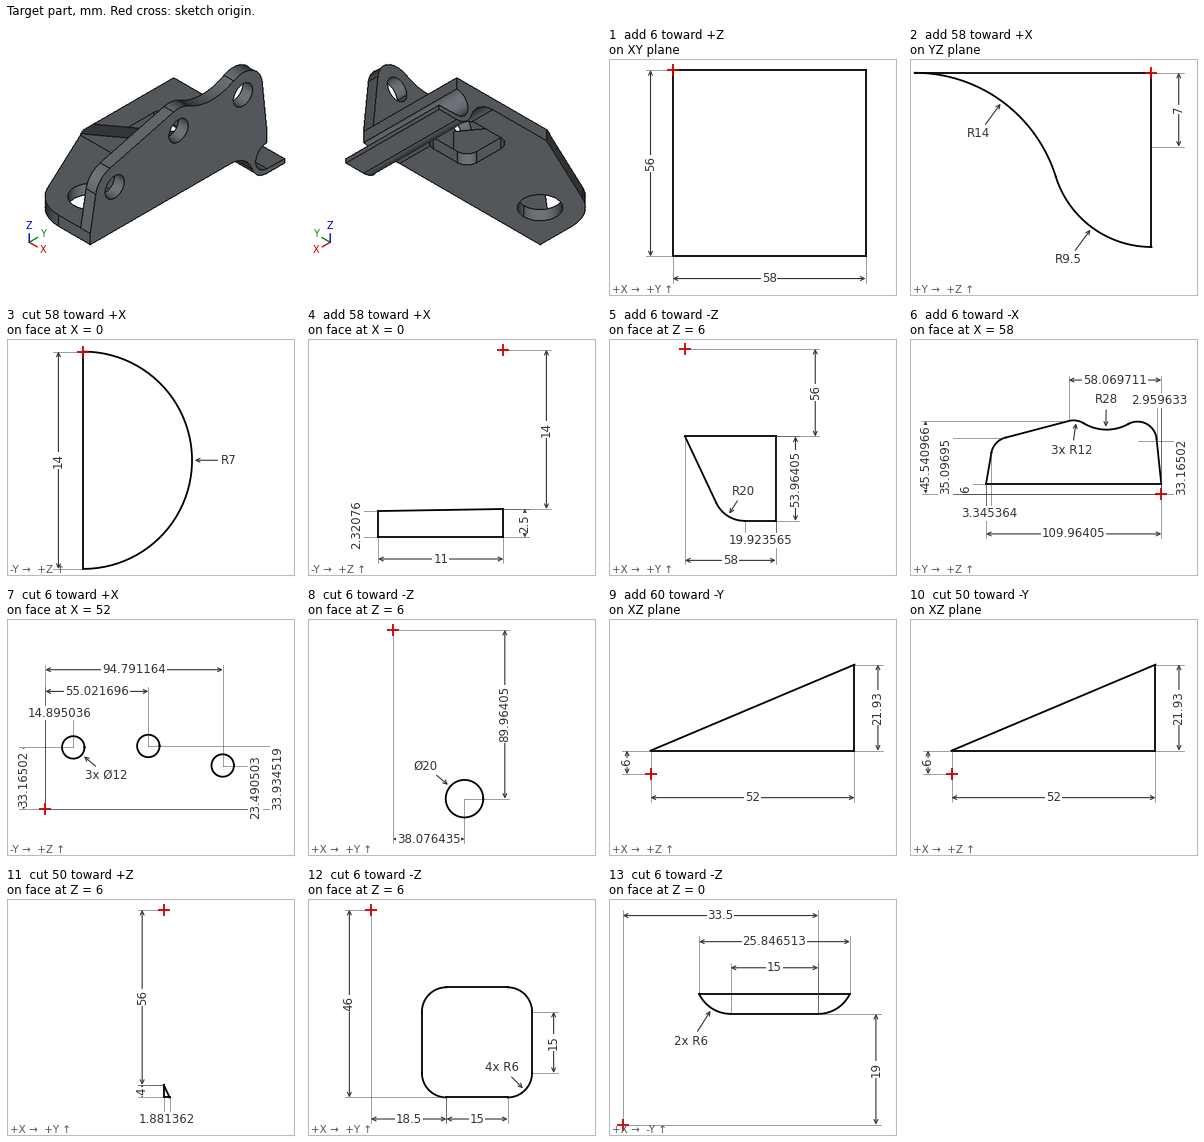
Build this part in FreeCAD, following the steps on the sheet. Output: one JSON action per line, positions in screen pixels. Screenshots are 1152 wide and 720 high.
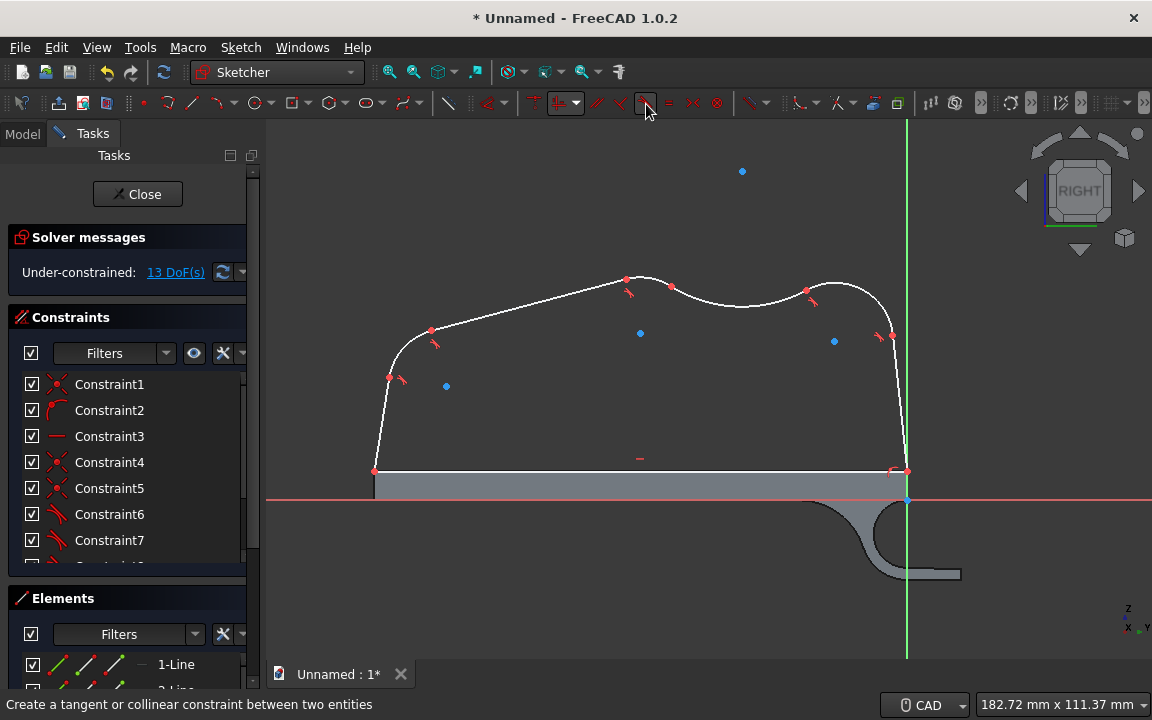
{"action": "left_click", "coordinate": [710, 303]}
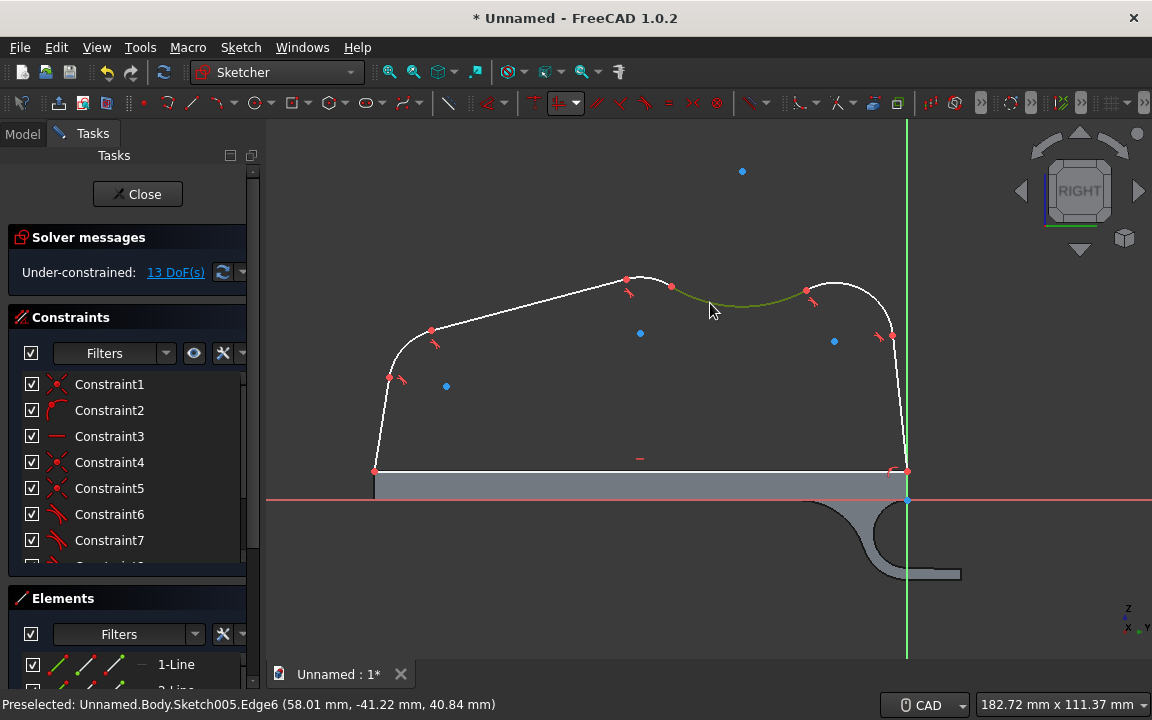
{"action": "left_click", "coordinate": [658, 280]}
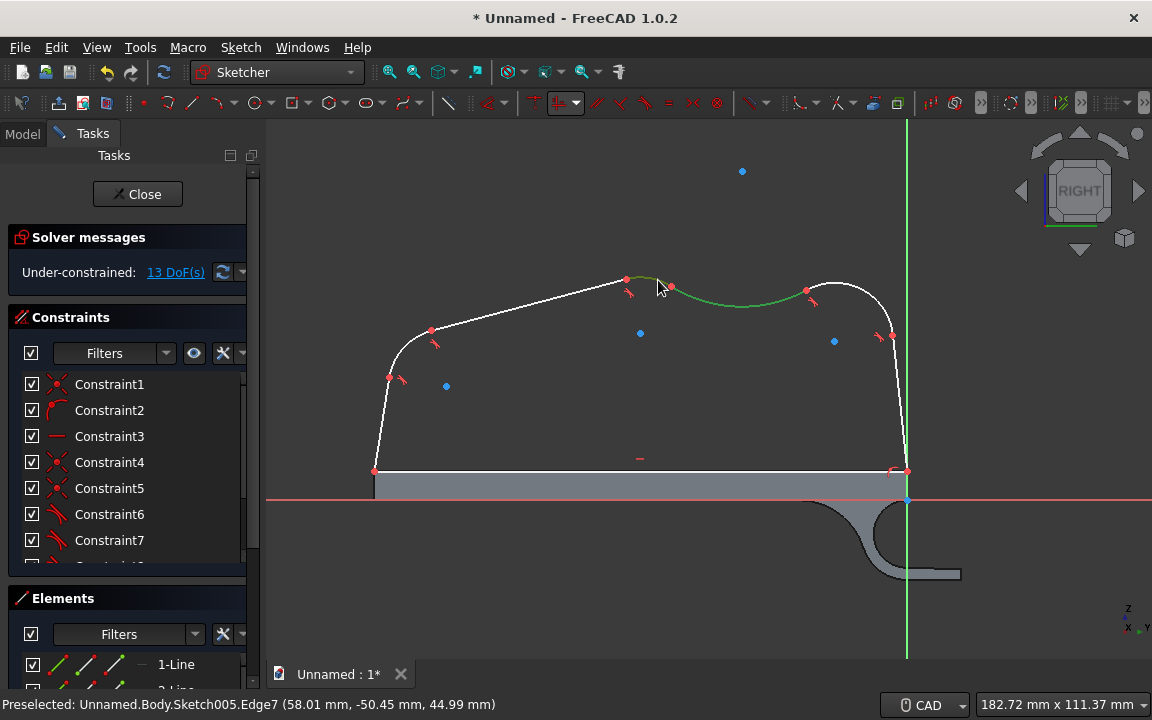
{"action": "key", "text": "t"}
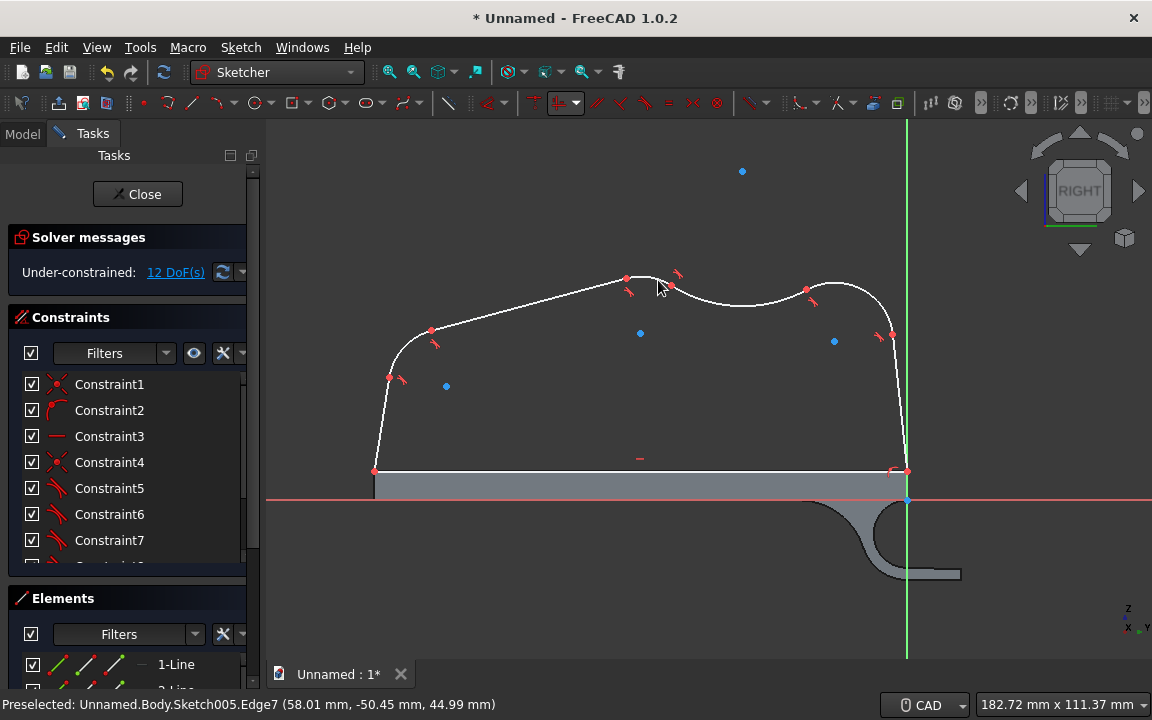
{"action": "left_click", "coordinate": [880, 304]}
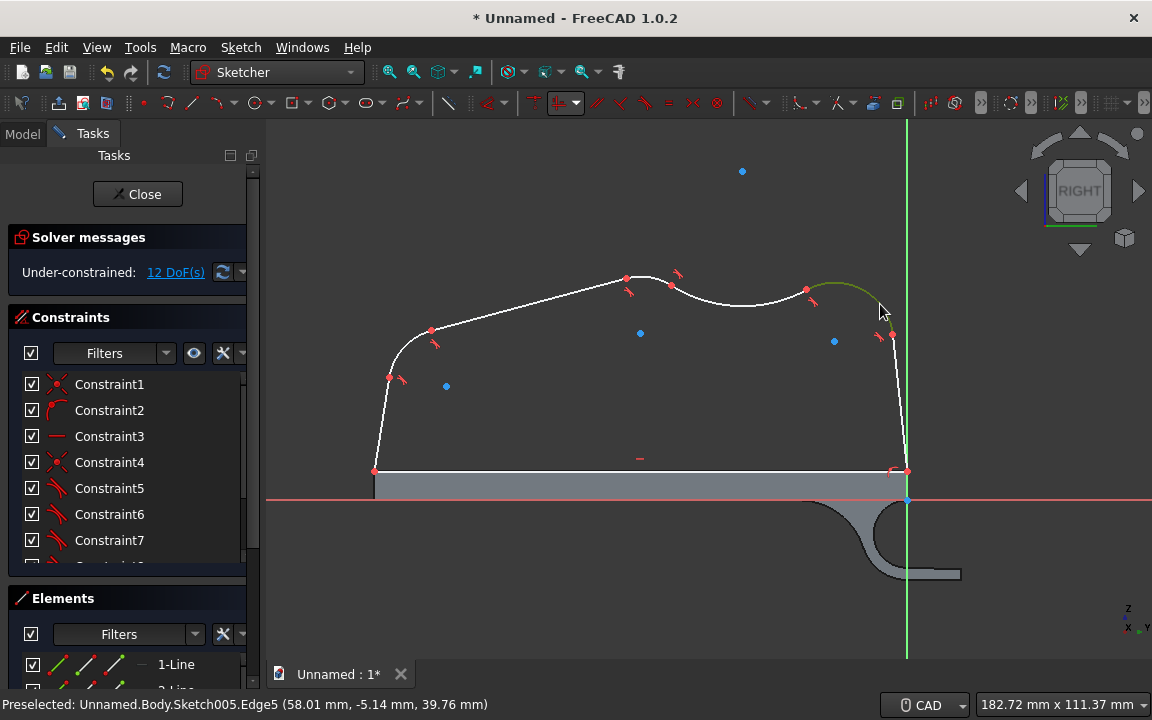
{"action": "left_click", "coordinate": [658, 279]}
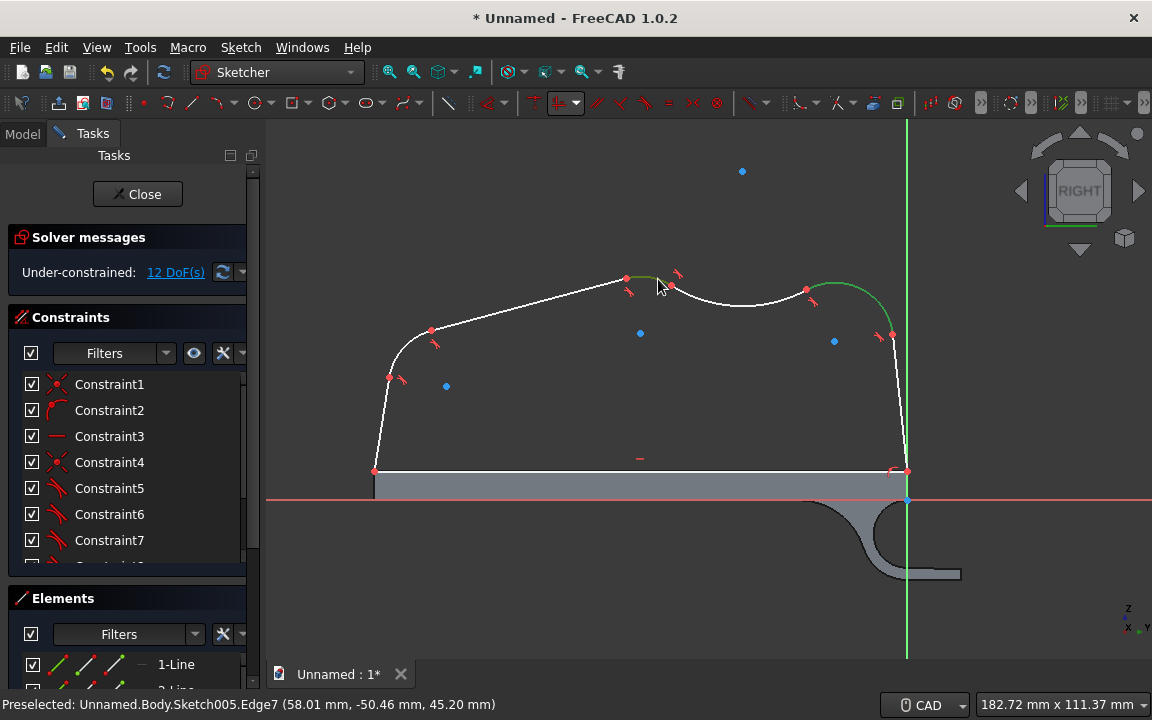
{"action": "left_click", "coordinate": [414, 339]}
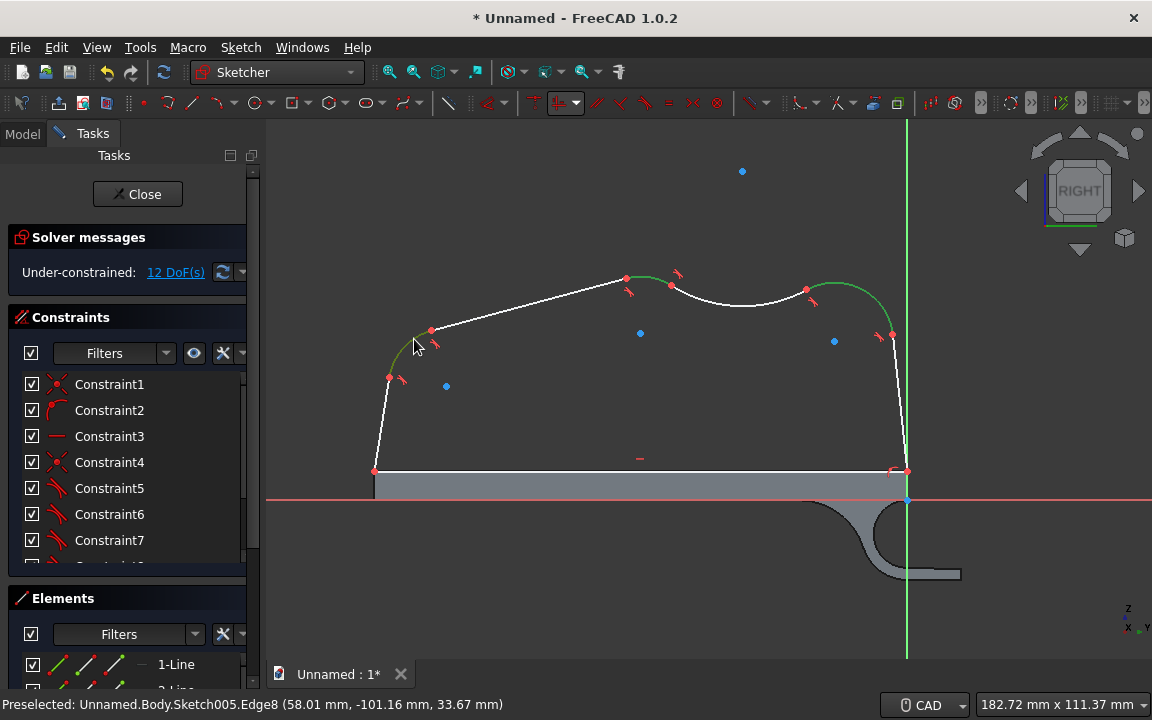
{"action": "left_click", "coordinate": [670, 104]}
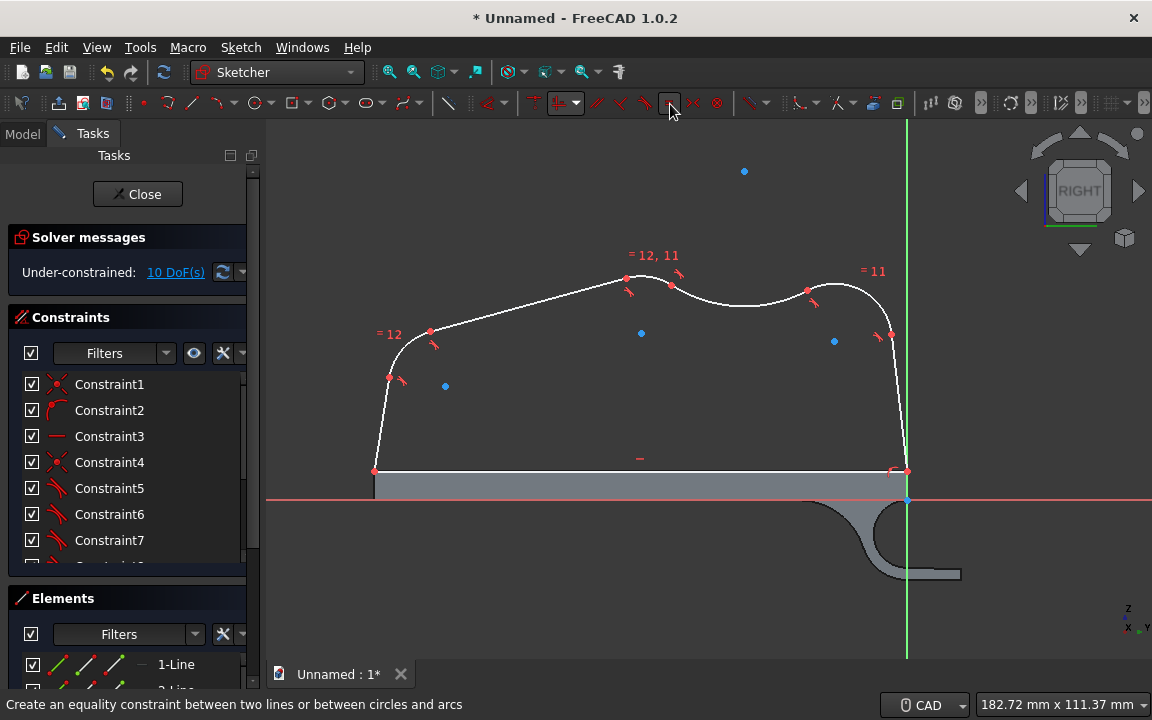
{"action": "left_click", "coordinate": [488, 104]}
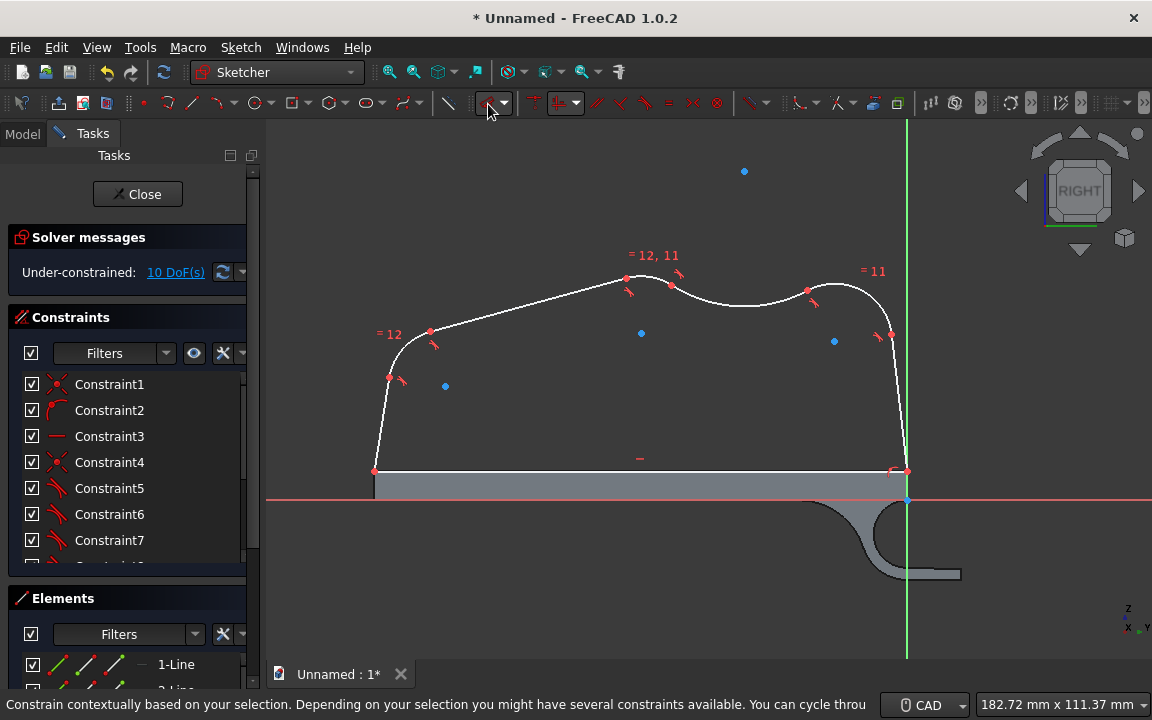
{"action": "left_click", "coordinate": [879, 304]}
{"action": "left_click", "coordinate": [923, 323]}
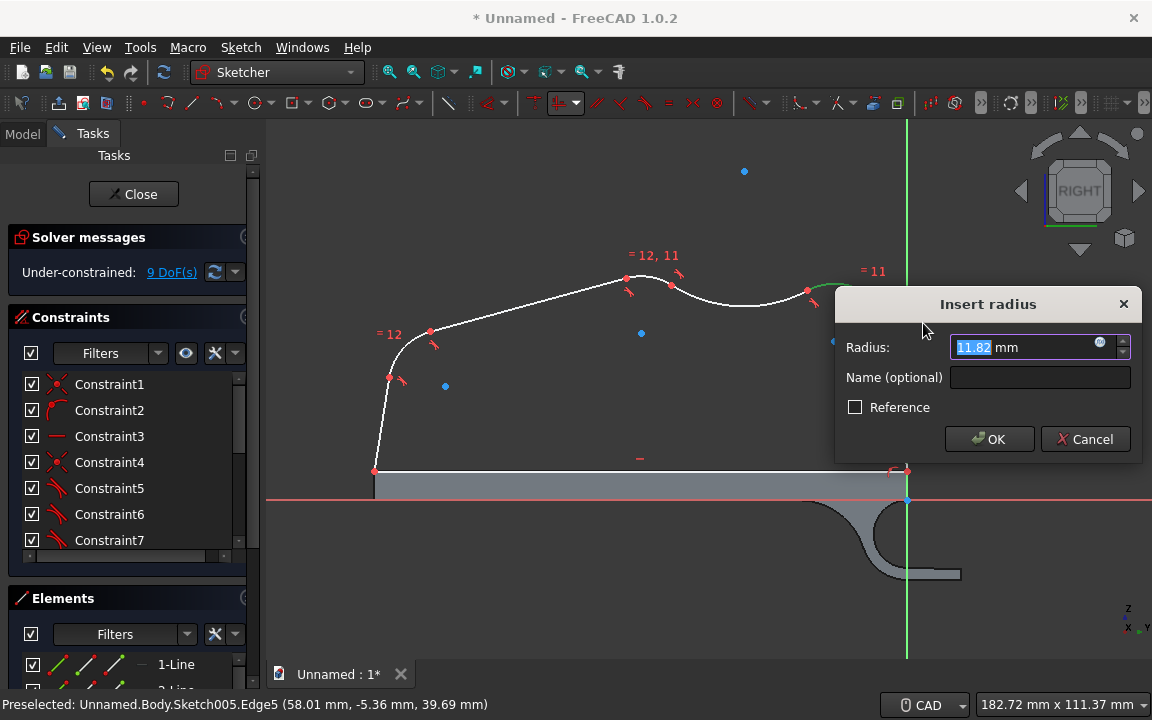
{"action": "type", "text": "12"}
{"action": "key", "text": "Return"}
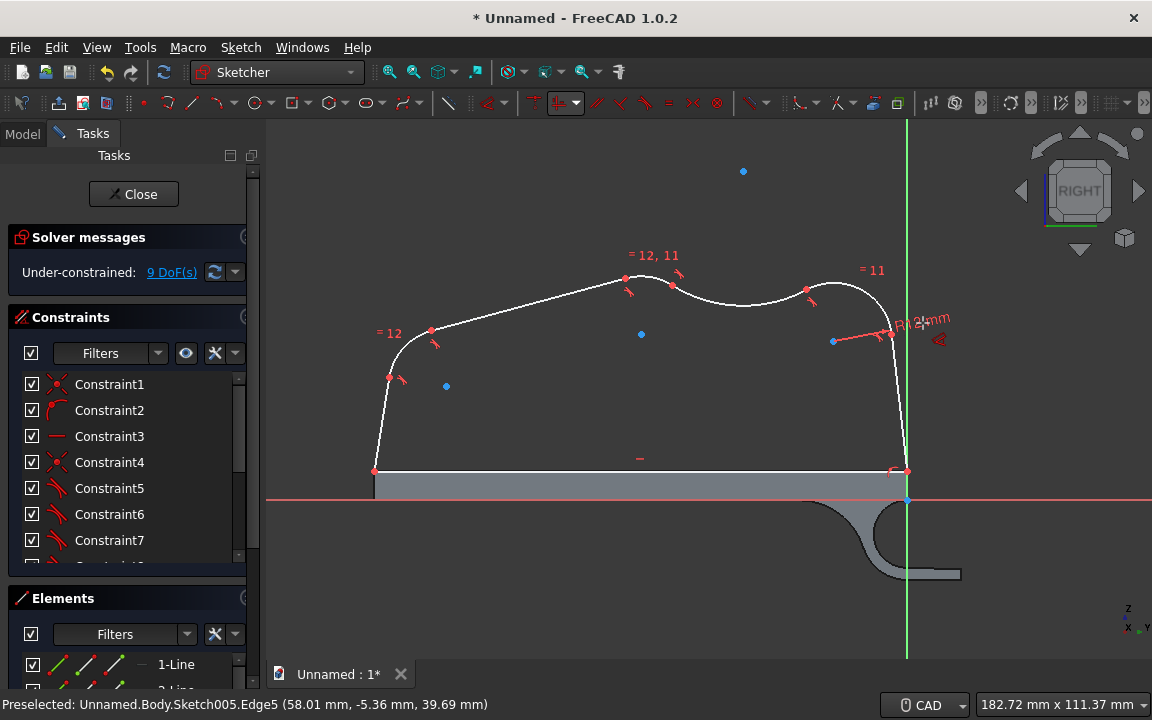
{"action": "left_click", "coordinate": [711, 302]}
{"action": "left_click", "coordinate": [703, 333]}